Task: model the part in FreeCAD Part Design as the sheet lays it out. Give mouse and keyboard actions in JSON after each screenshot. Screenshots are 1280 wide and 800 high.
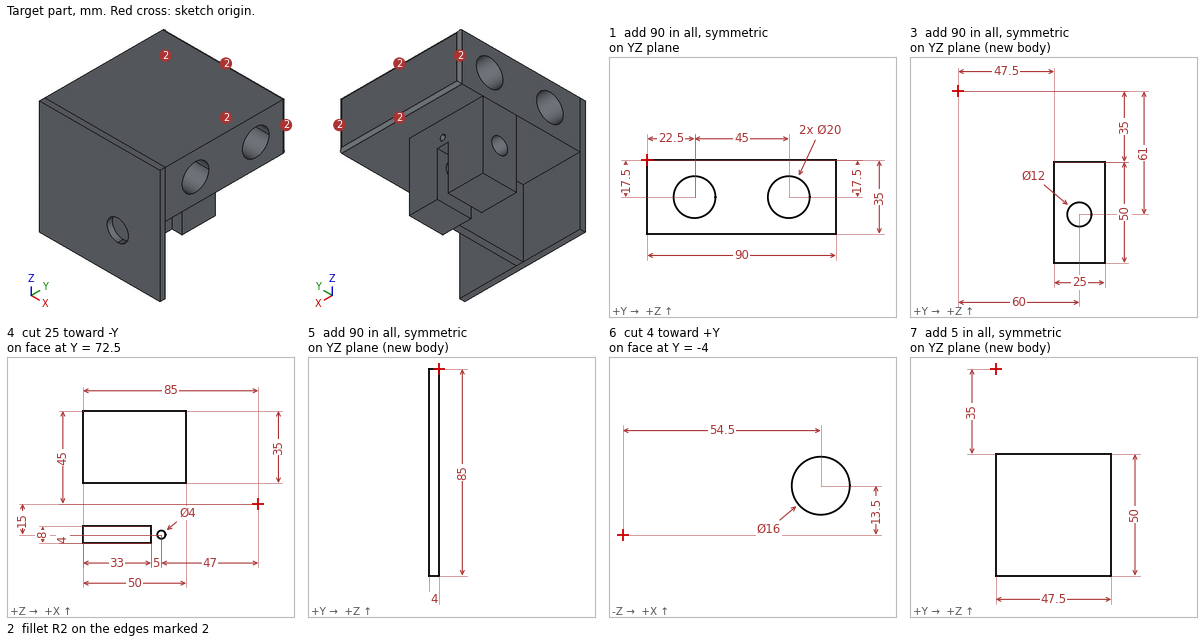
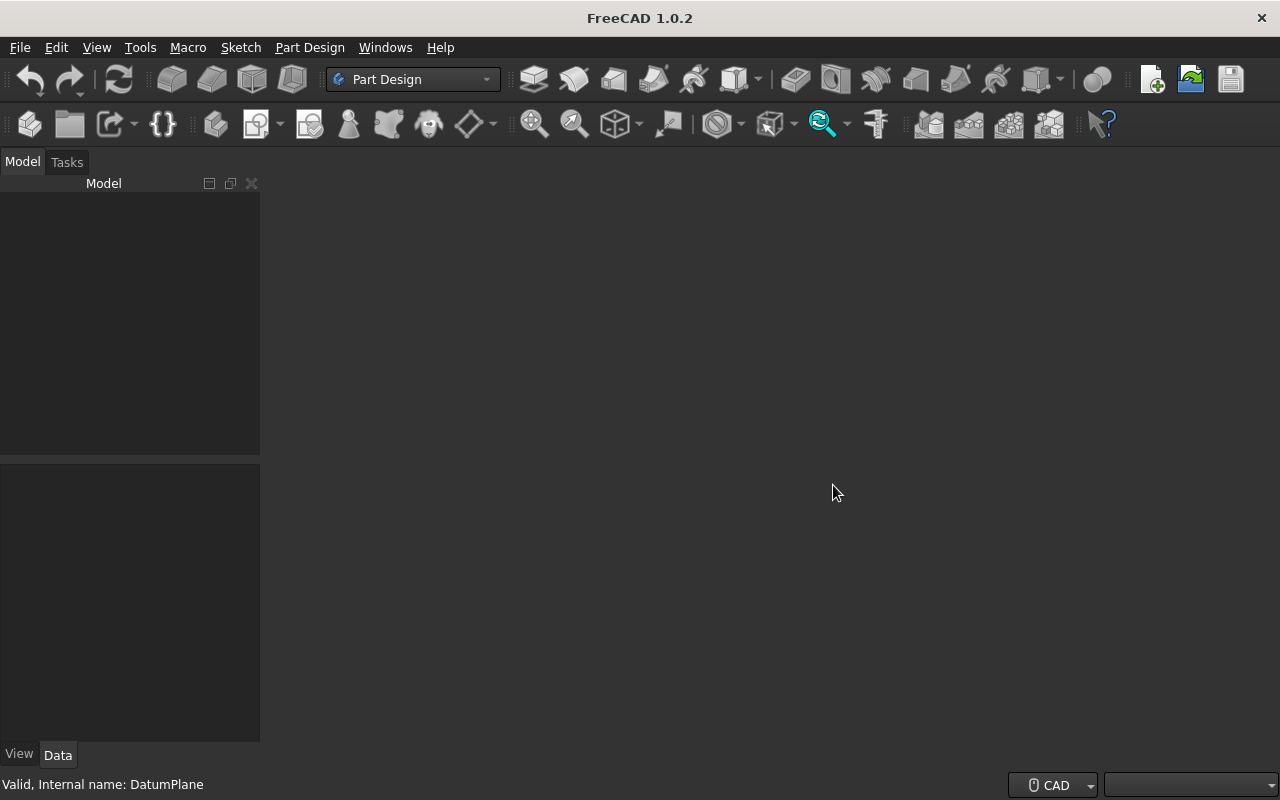
{"action": "left_click", "coordinate": [1152, 80]}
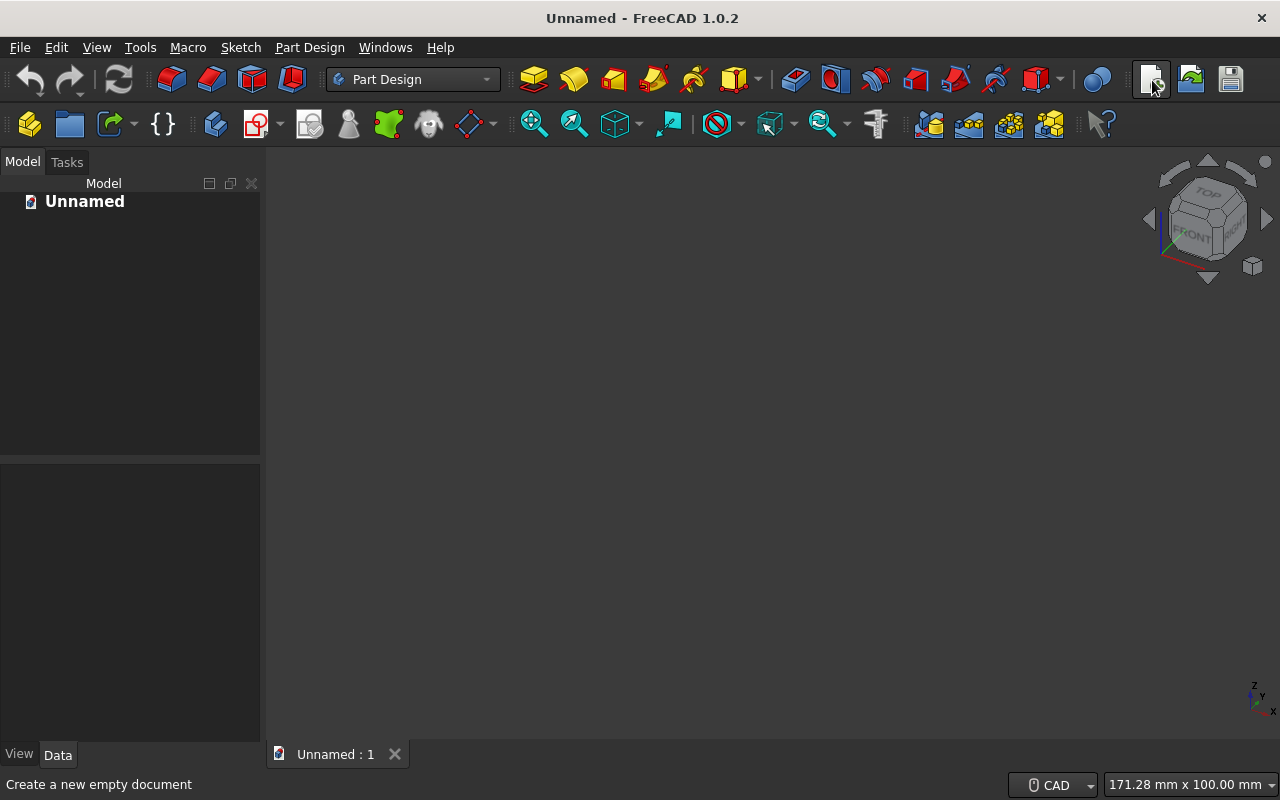
{"action": "left_click", "coordinate": [256, 124]}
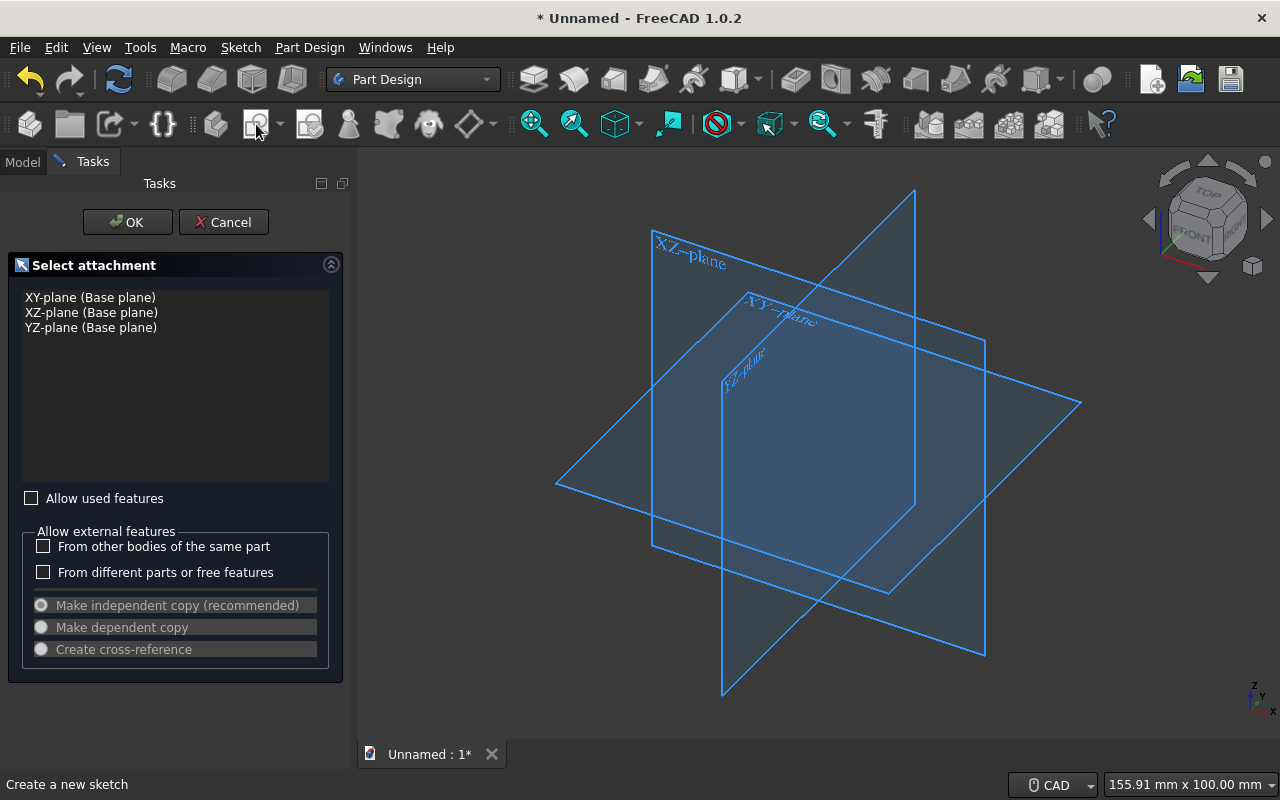
{"action": "left_click", "coordinate": [82, 328]}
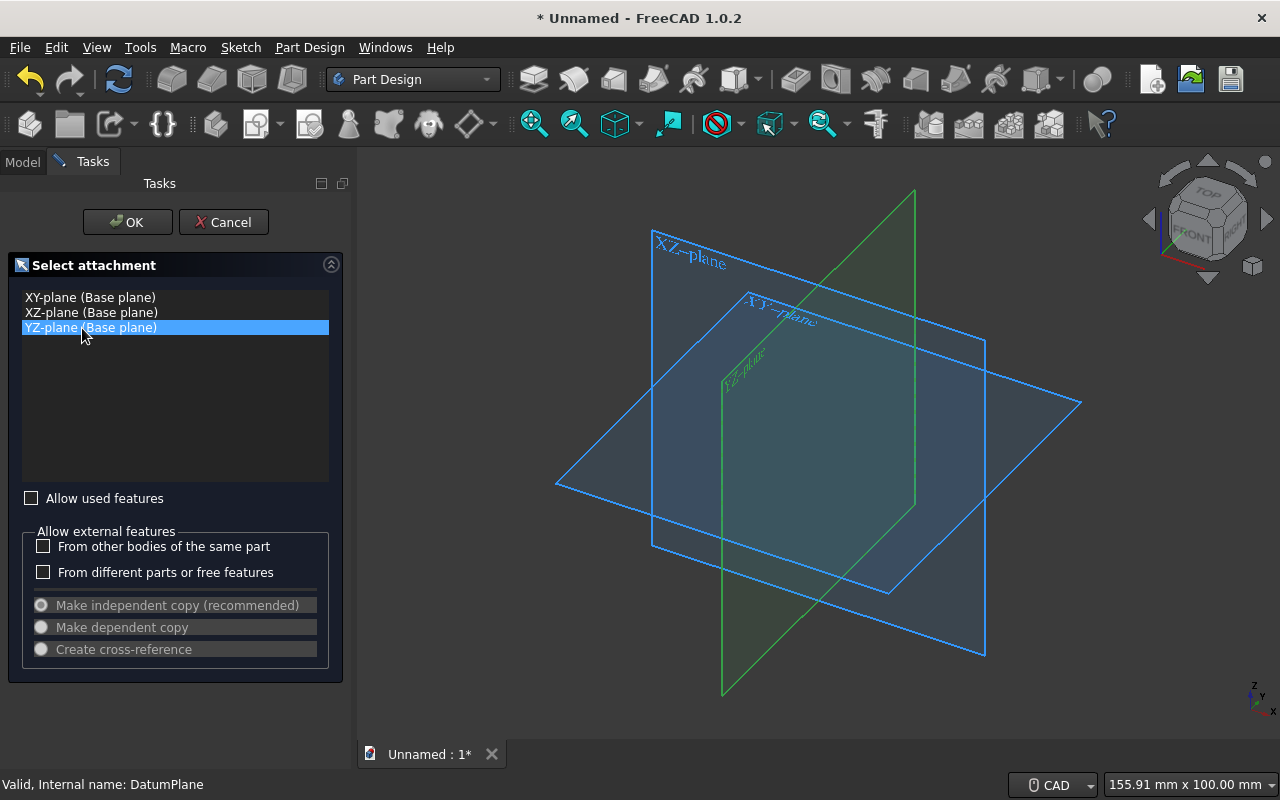
{"action": "left_click", "coordinate": [128, 222]}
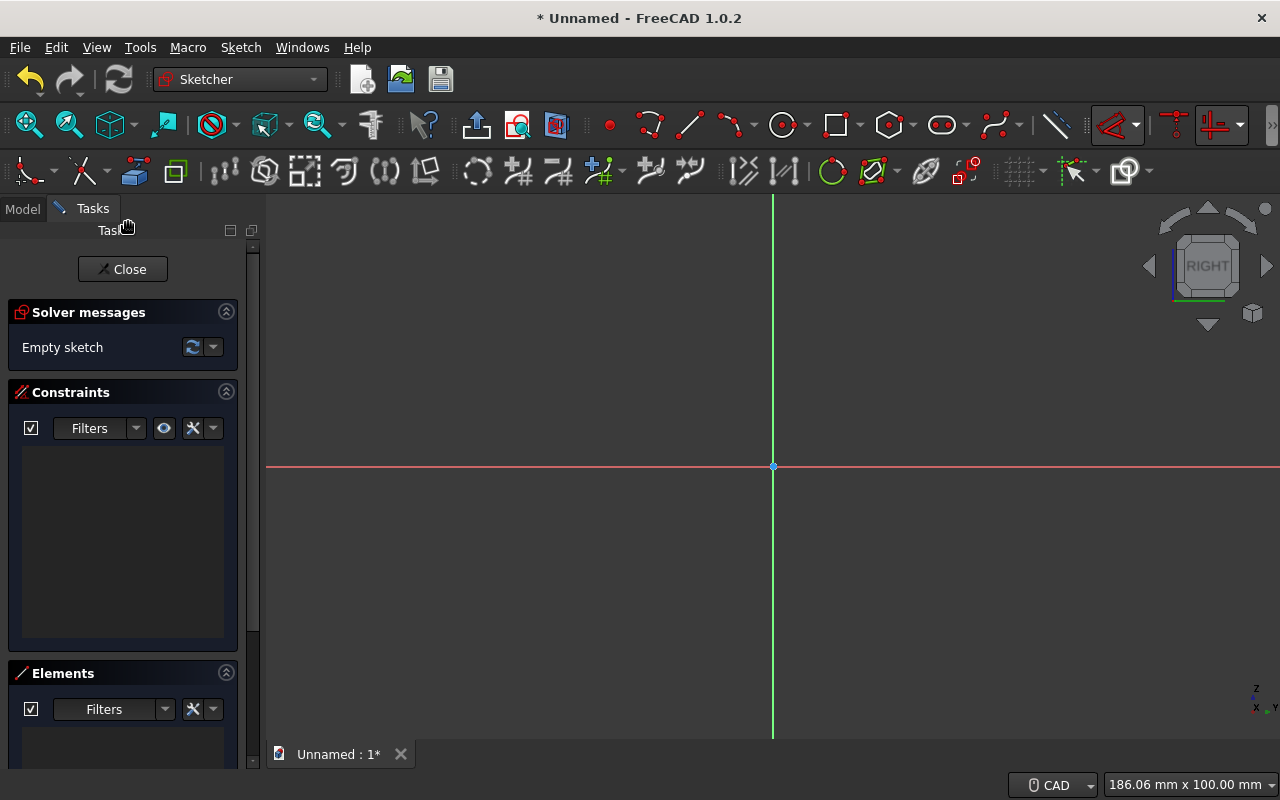
{"action": "scroll", "coordinate": [294, 222], "scroll_direction": "down", "scroll_amount": 1}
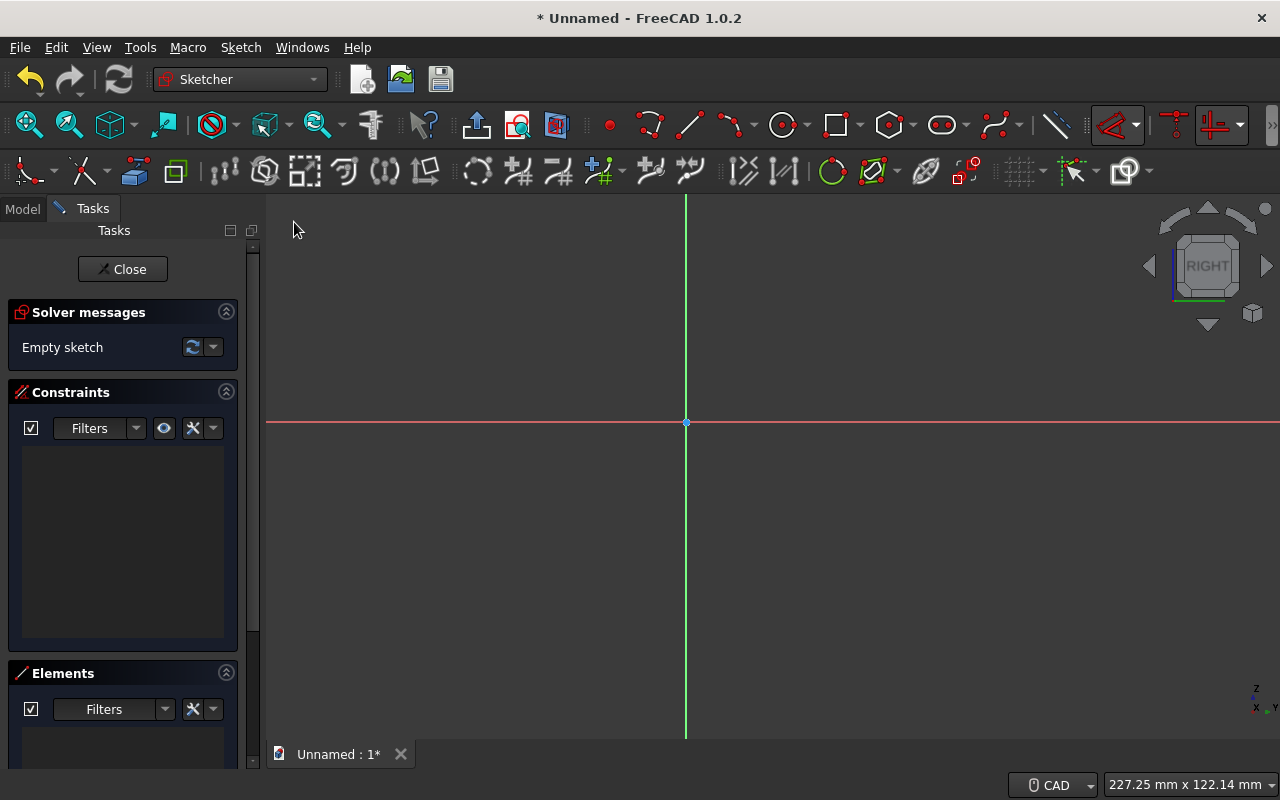
{"action": "scroll", "coordinate": [1115, 569], "scroll_direction": "up", "scroll_amount": 2}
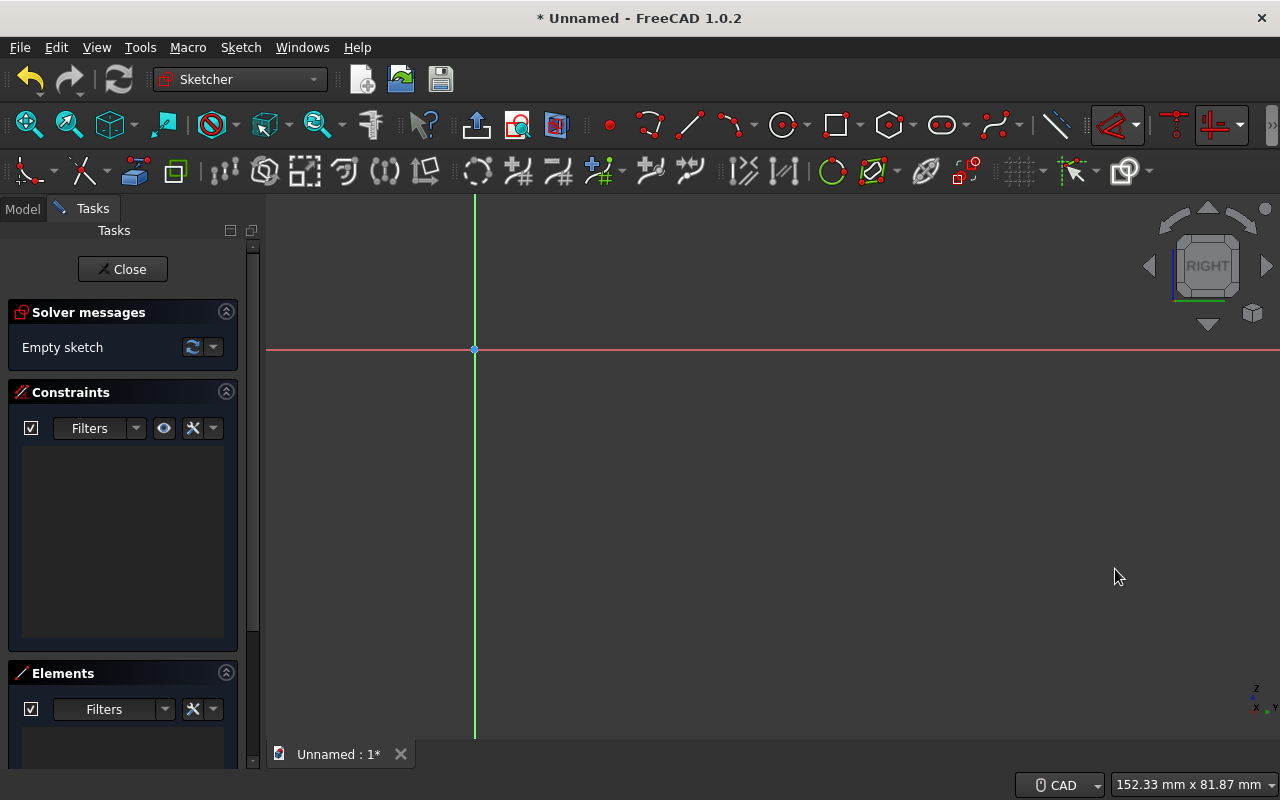
{"action": "left_click", "coordinate": [836, 126]}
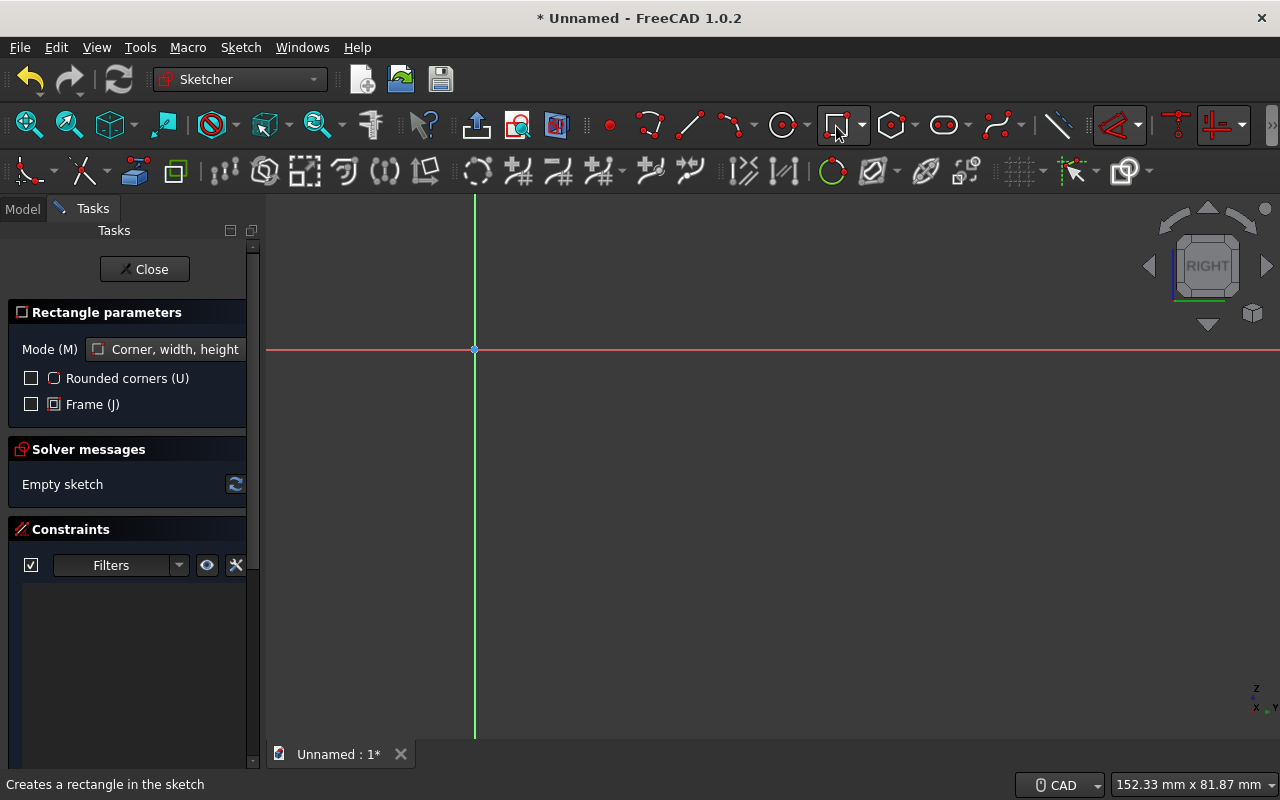
{"action": "left_click", "coordinate": [475, 350]}
{"action": "mouse_move", "coordinate": [1074, 583]}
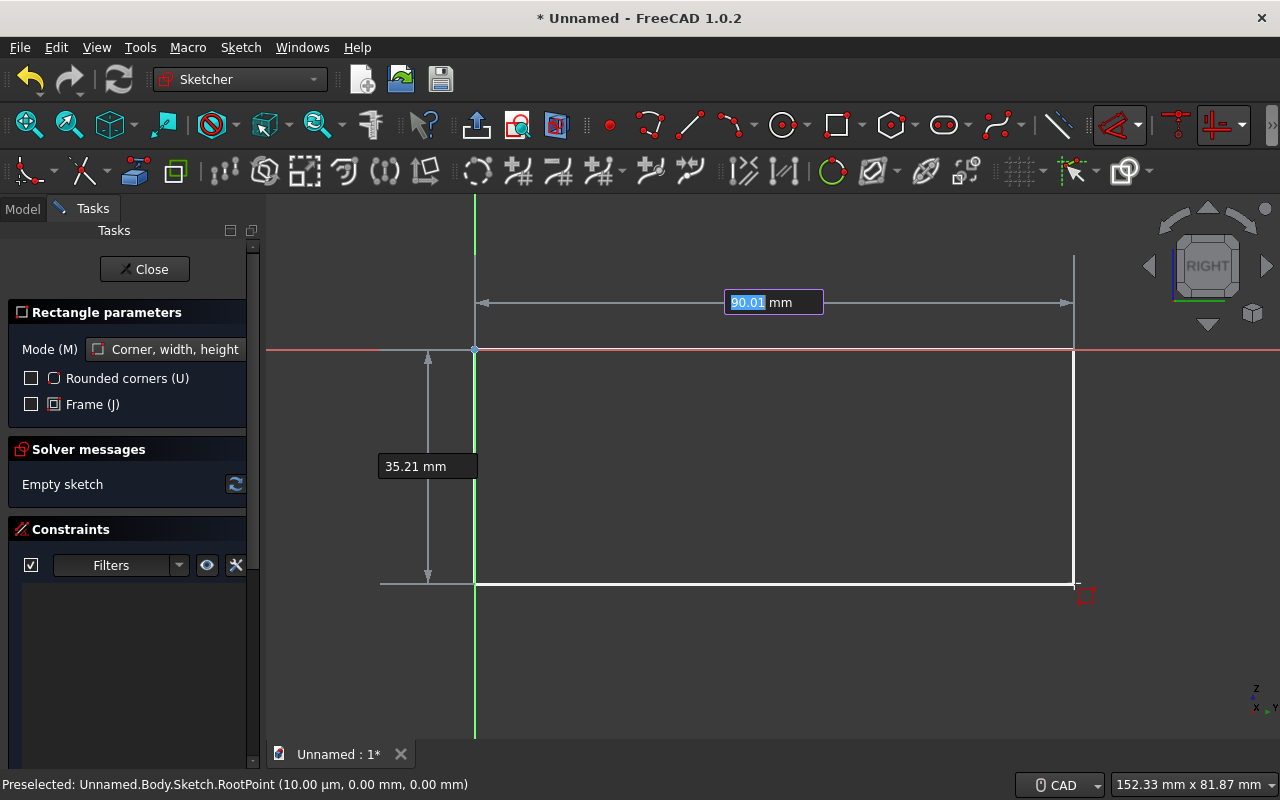
{"action": "type", "text": "90"}
{"action": "key", "text": "Tab"}
{"action": "type", "text": "35"}
{"action": "key", "text": "Return"}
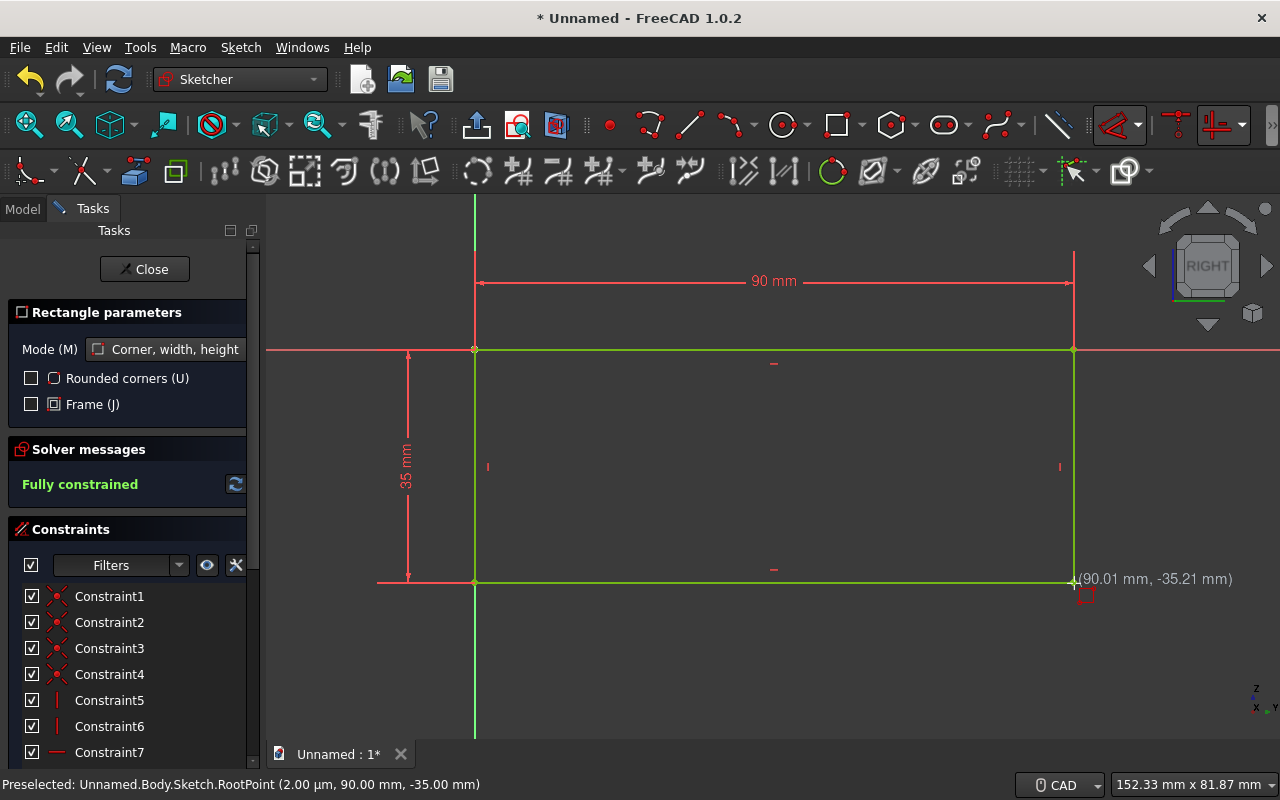
{"action": "left_click", "coordinate": [784, 126]}